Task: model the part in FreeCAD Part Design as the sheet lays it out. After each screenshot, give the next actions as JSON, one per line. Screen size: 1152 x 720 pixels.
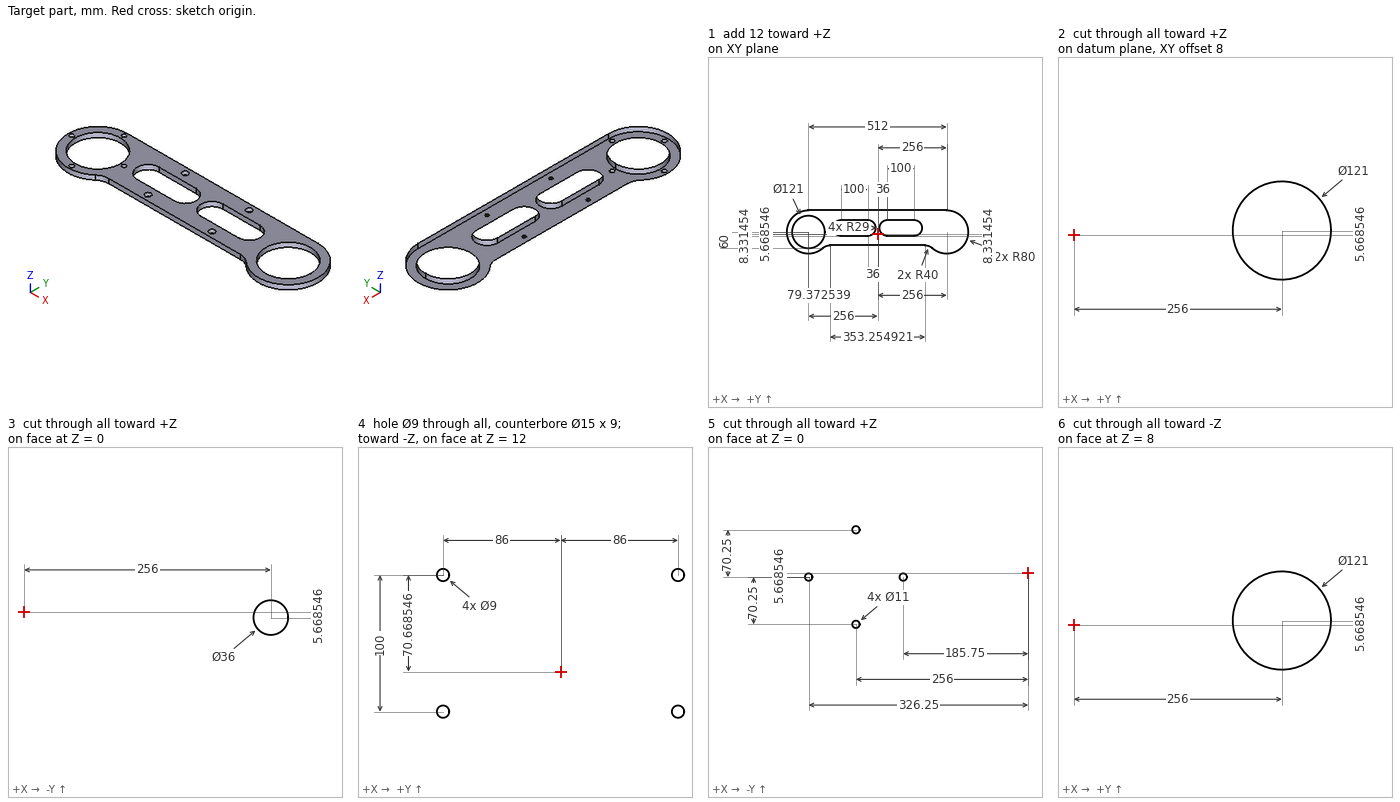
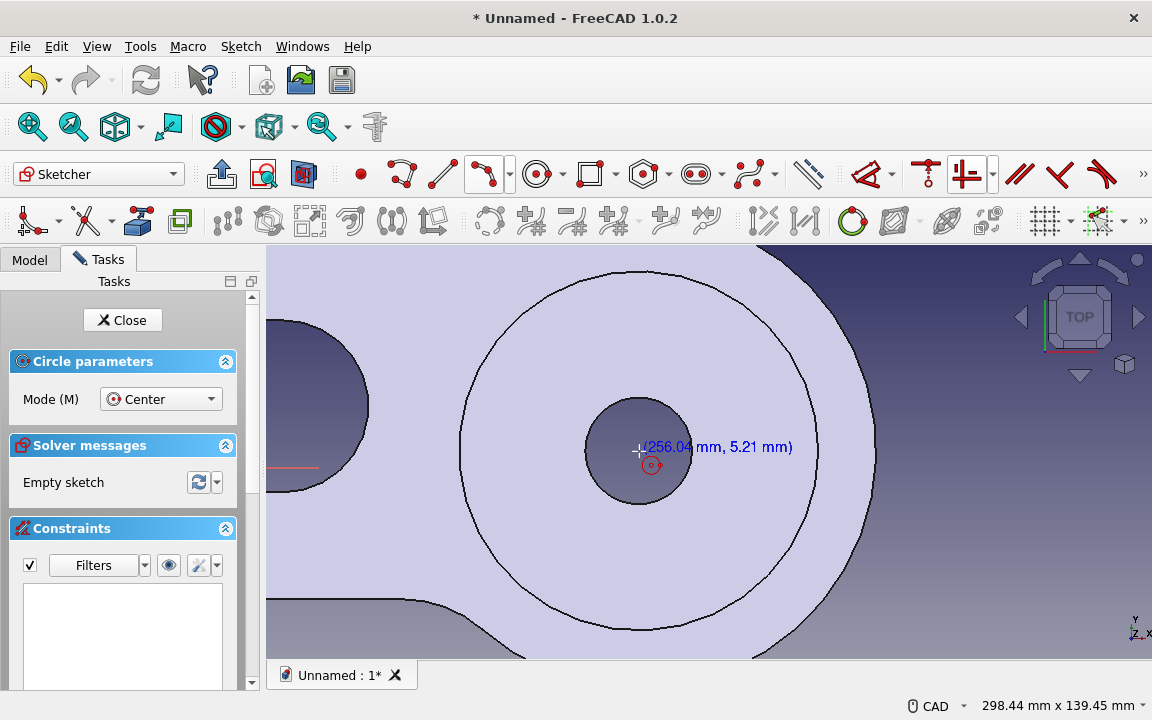
{"action": "left_click", "coordinate": [639, 451]}
{"action": "mouse_move", "coordinate": [766, 324]}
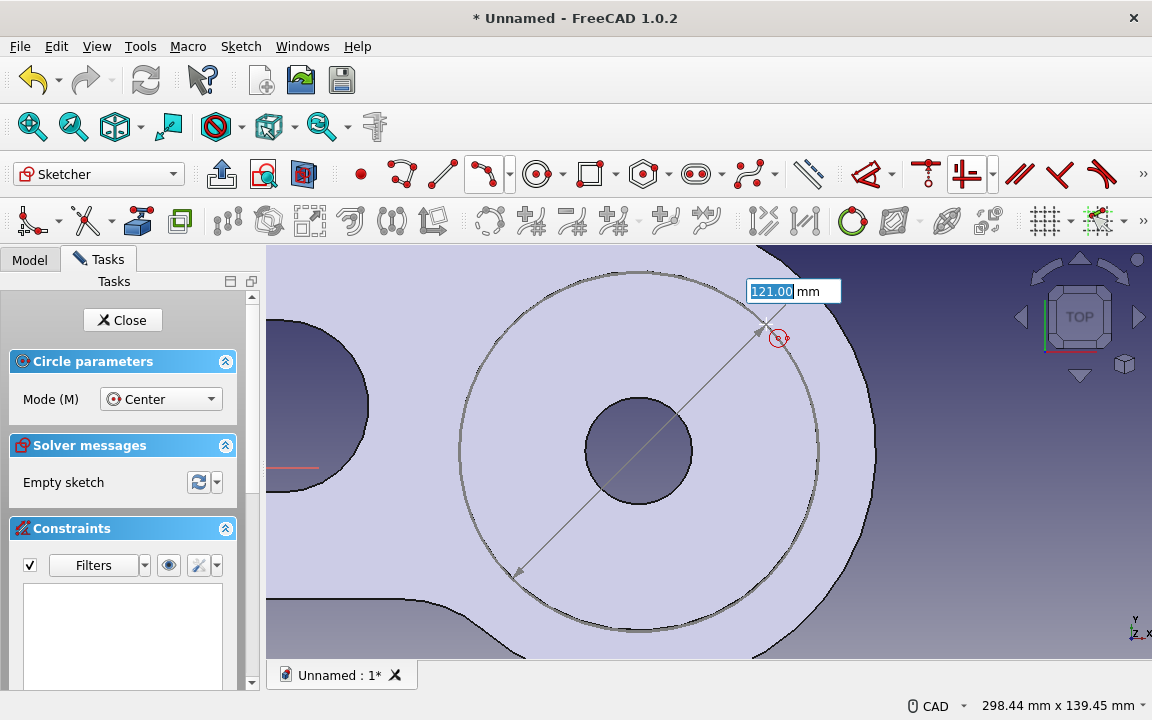
{"action": "type", "text": "121"}
{"action": "key", "text": "Return"}
{"action": "key", "text": "Escape"}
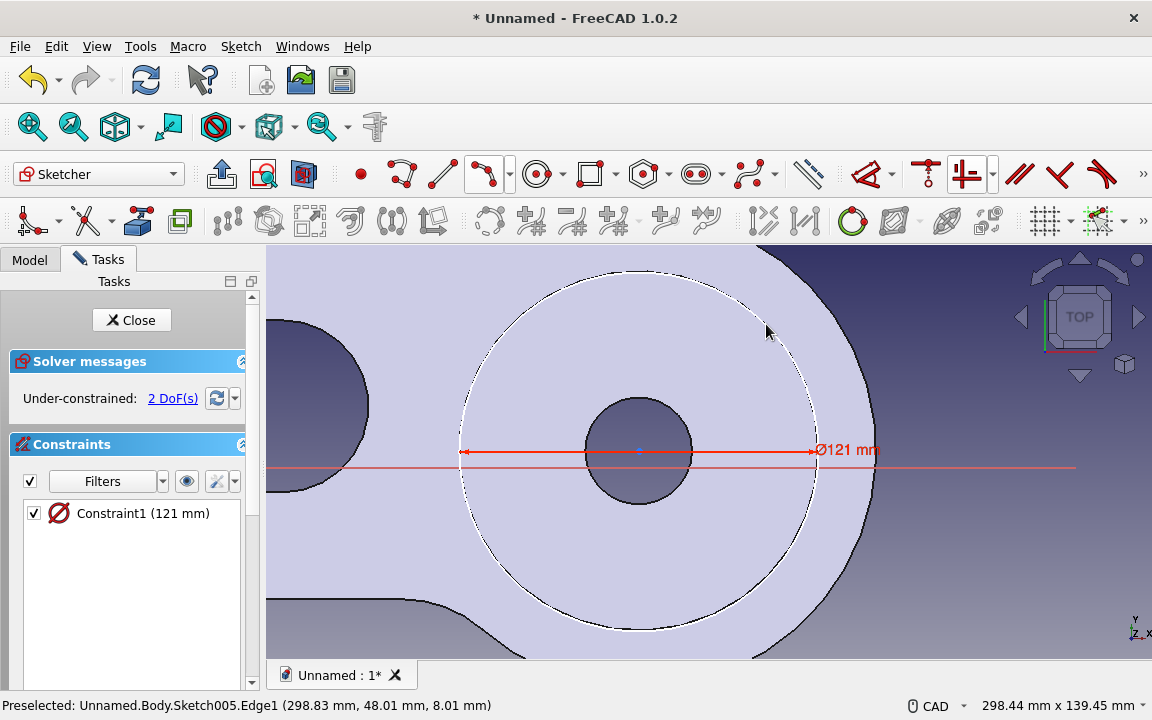
{"action": "left_click", "coordinate": [866, 174]}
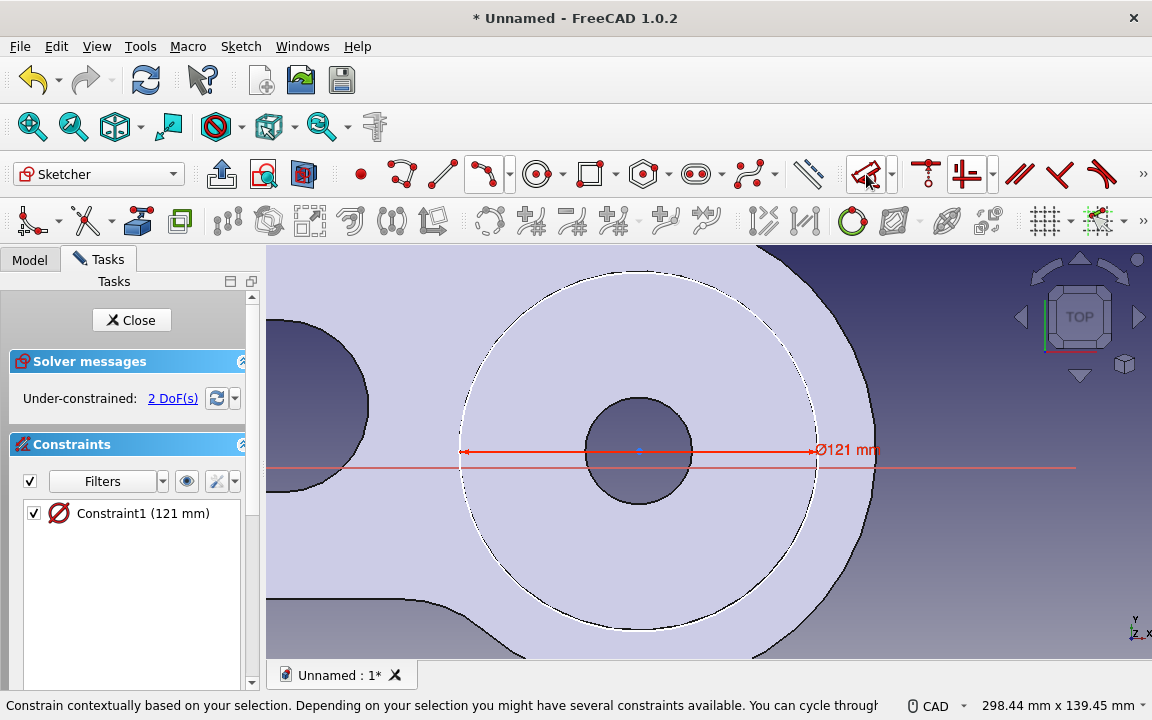
{"action": "left_click", "coordinate": [639, 452]}
{"action": "left_click", "coordinate": [387, 502]}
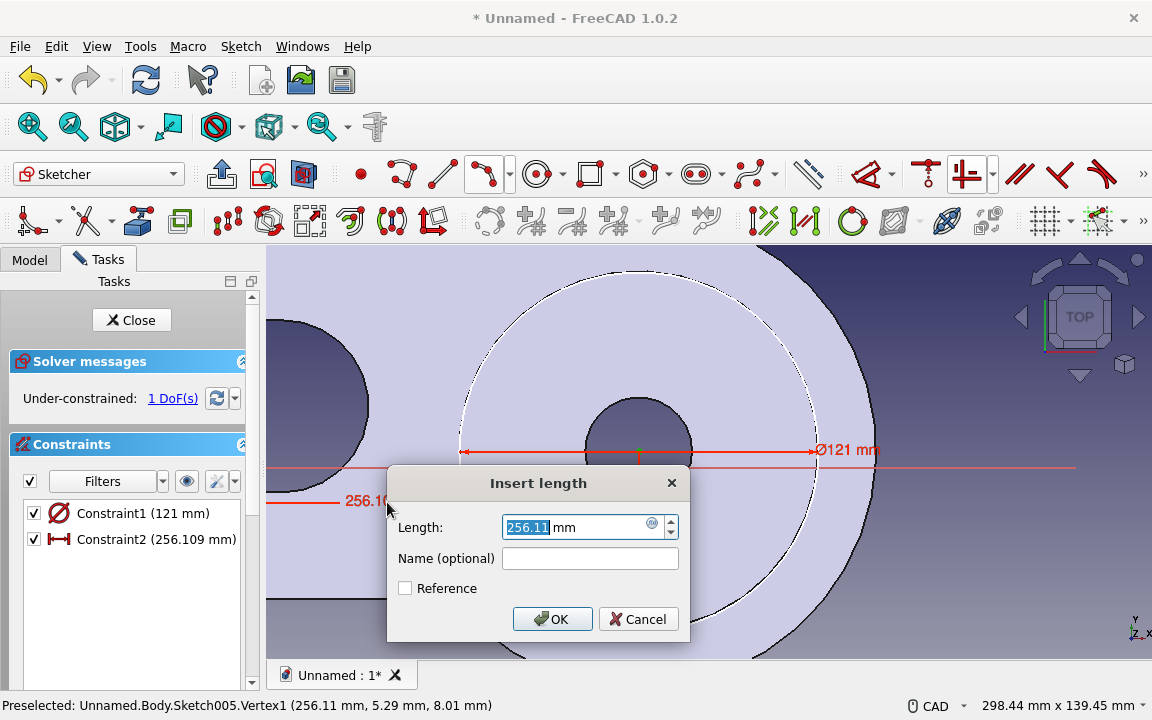
{"action": "type", "text": "256"}
{"action": "key", "text": "Return"}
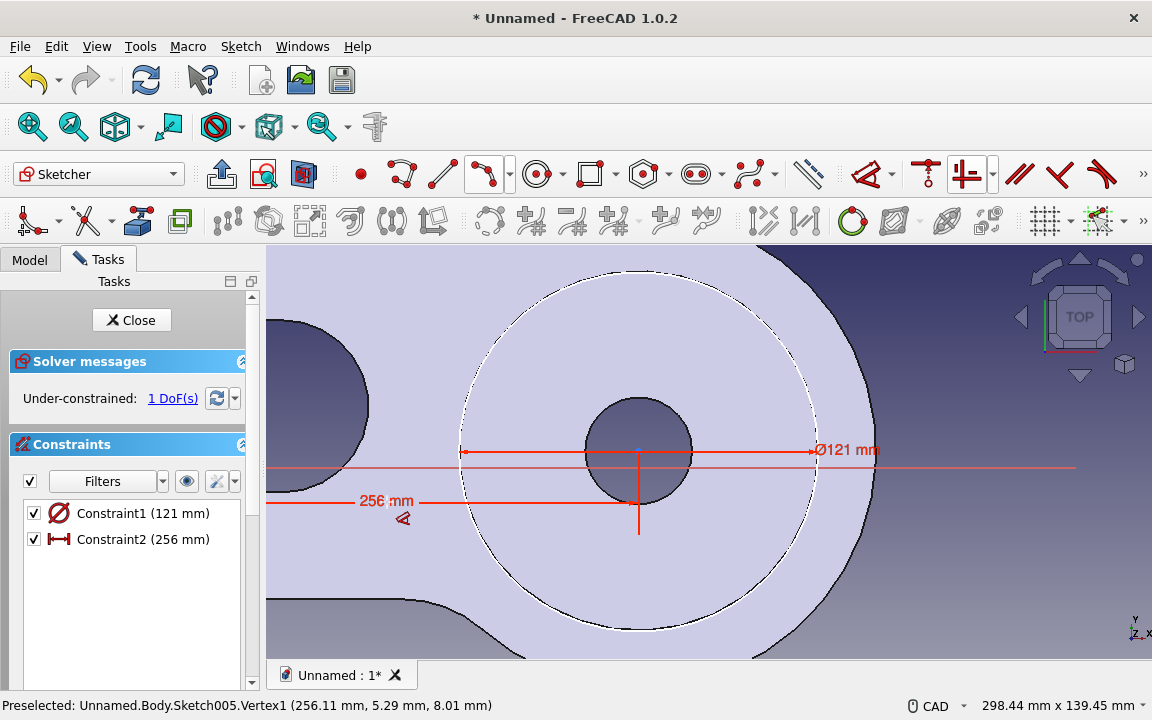
{"action": "scroll", "coordinate": [639, 452], "scroll_direction": "up", "scroll_amount": 5}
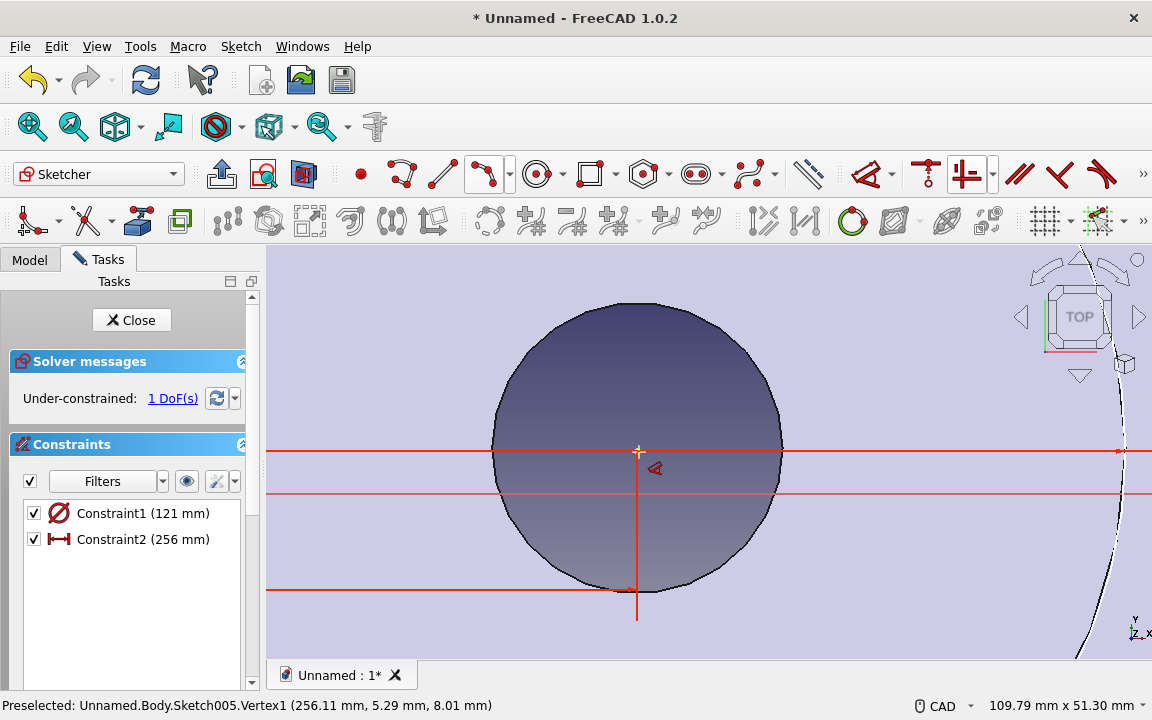
{"action": "left_click", "coordinate": [637, 451]}
{"action": "left_click", "coordinate": [671, 472]}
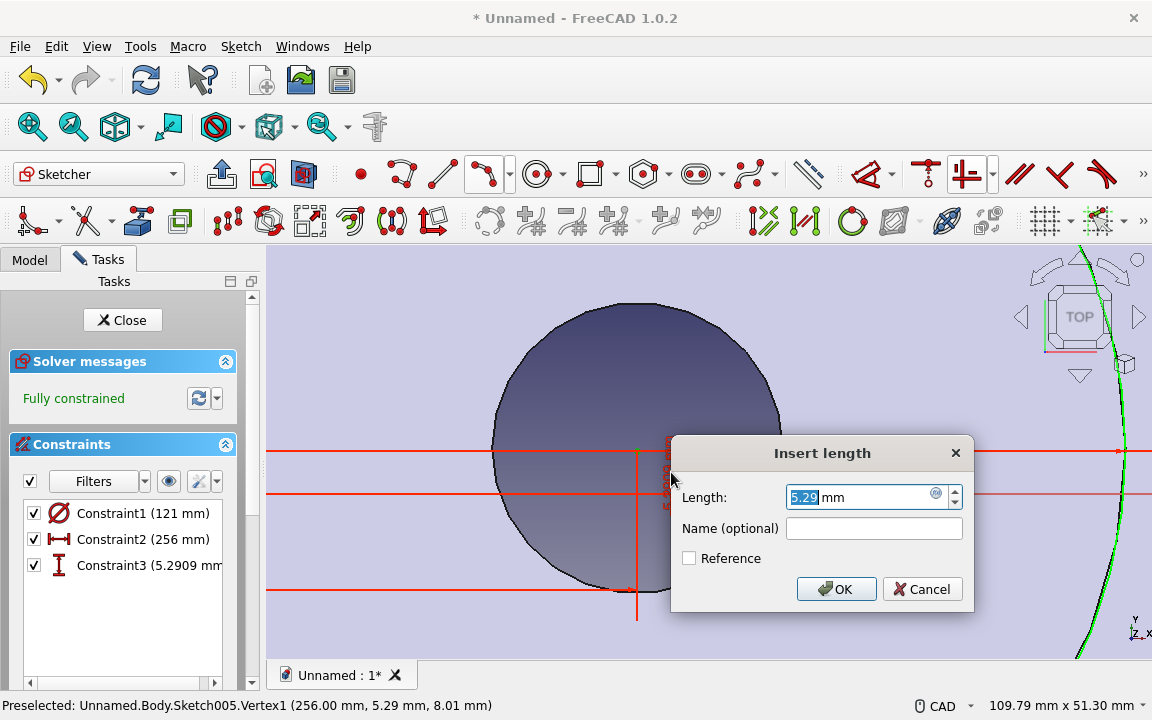
{"action": "type", "text": "5.668546"}
{"action": "key", "text": "Return"}
{"action": "key", "text": "Escape"}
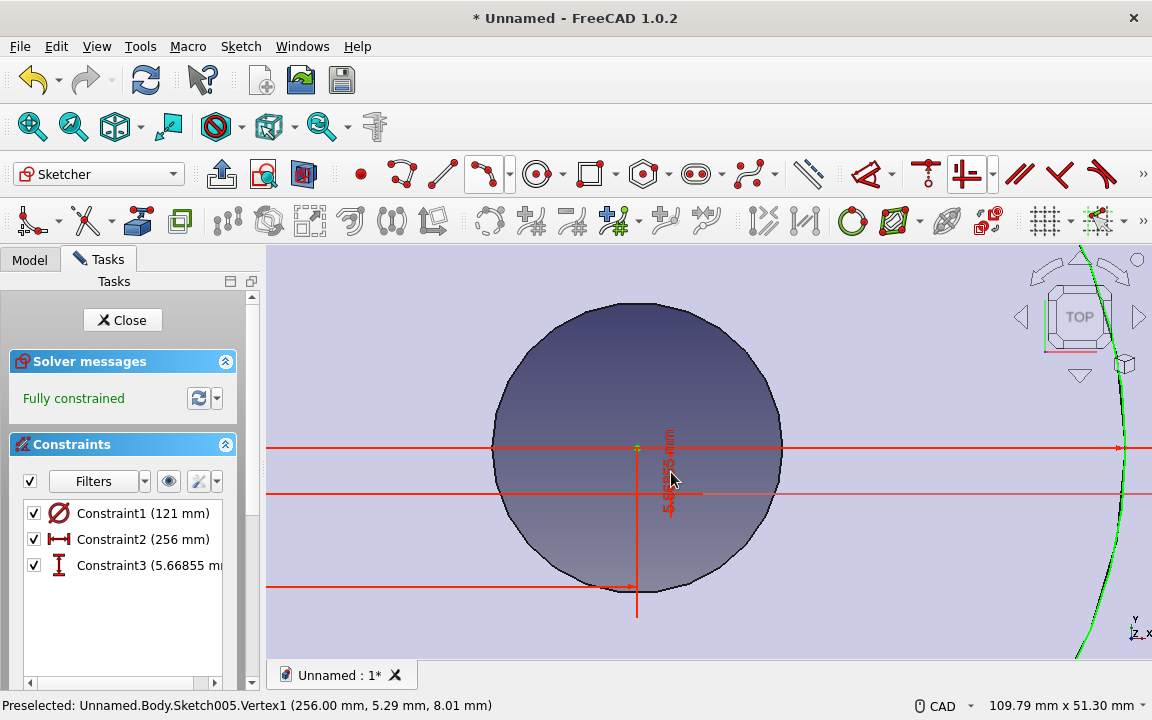
{"action": "left_click", "coordinate": [123, 320]}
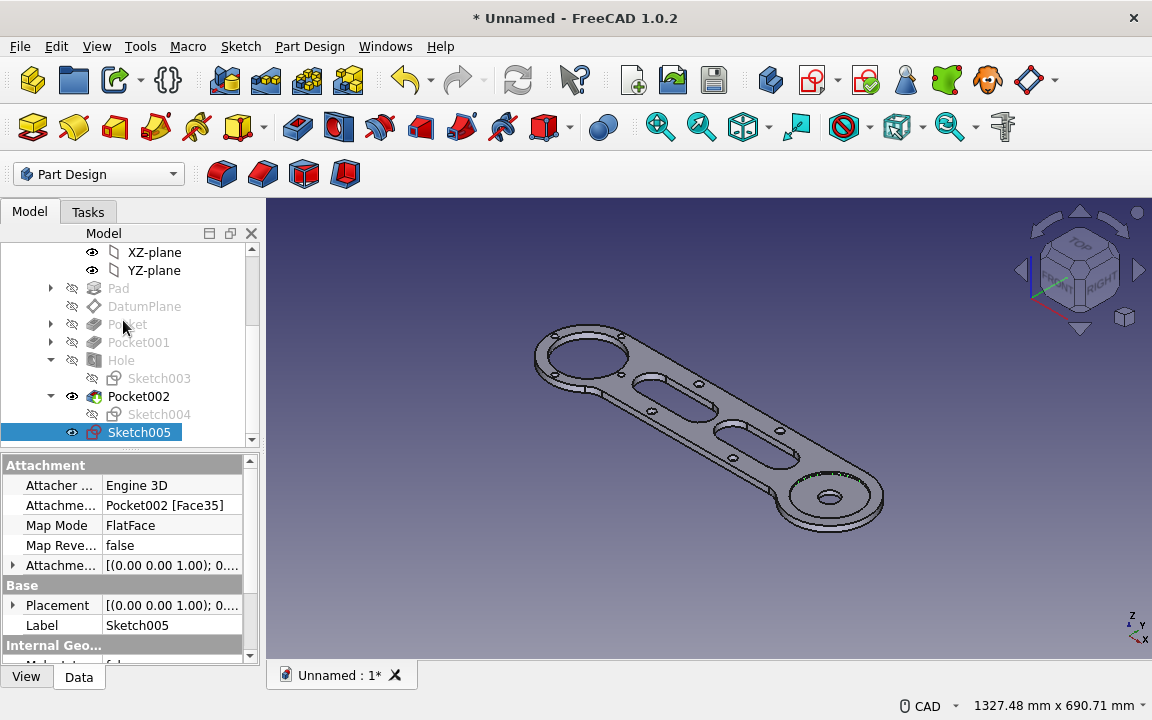
{"action": "left_click", "coordinate": [298, 128]}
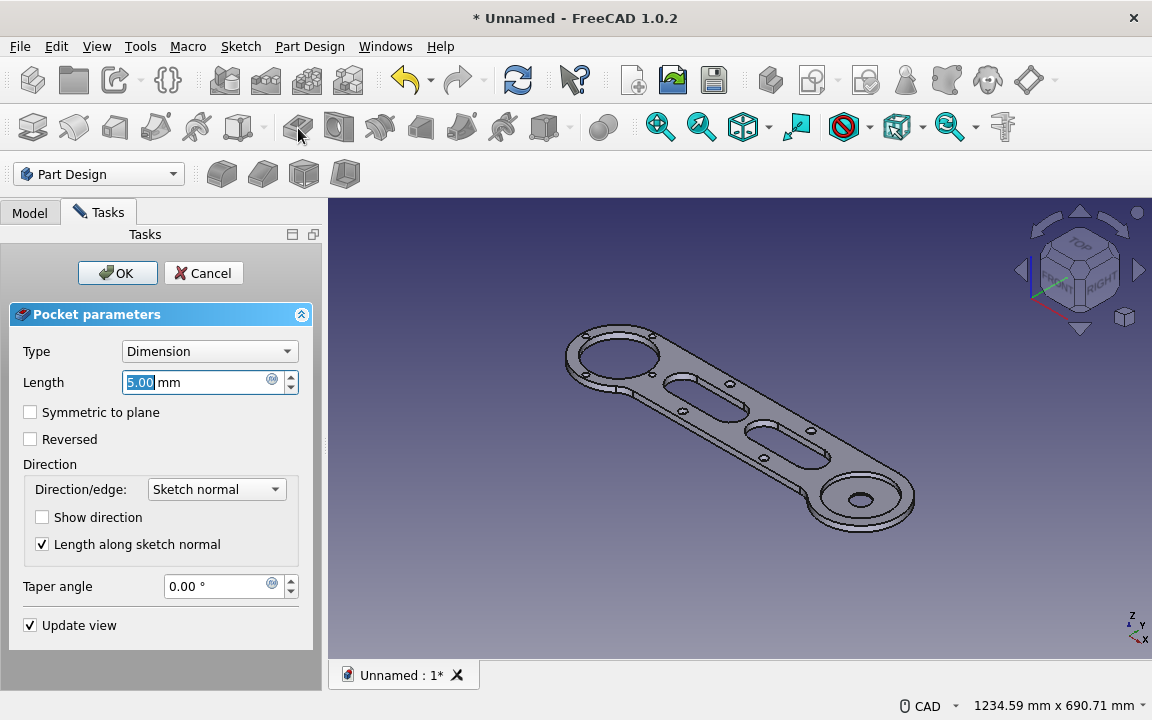
{"action": "left_click", "coordinate": [210, 352]}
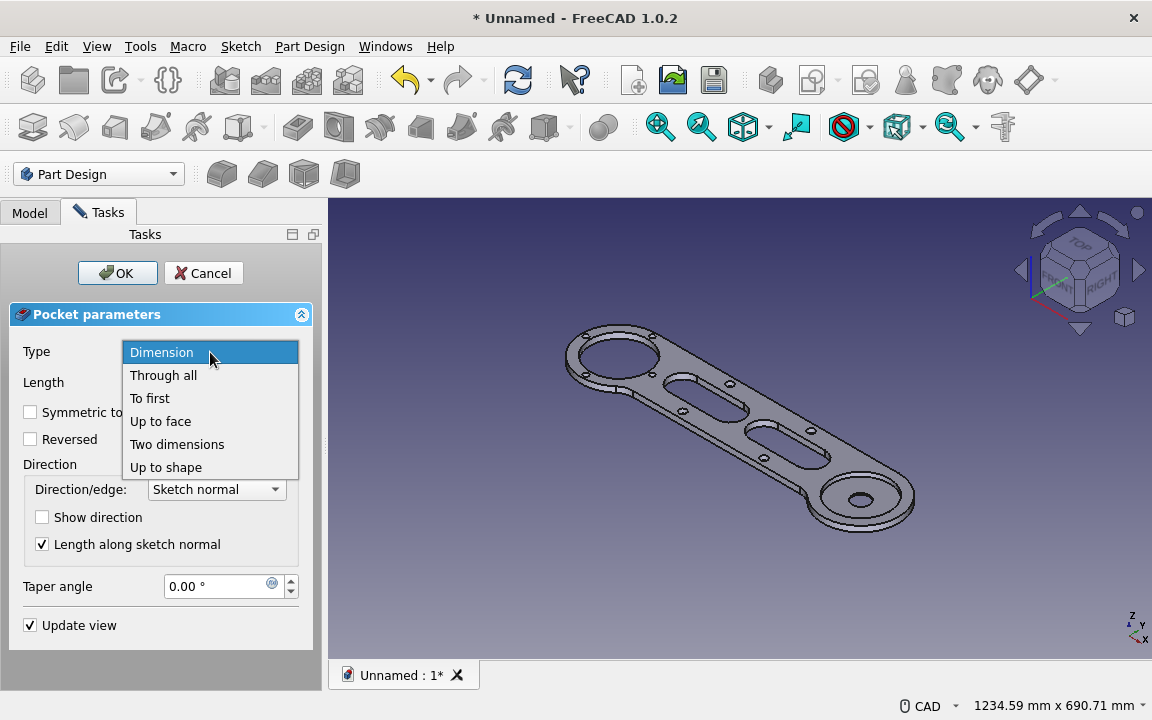
{"action": "left_click", "coordinate": [208, 376]}